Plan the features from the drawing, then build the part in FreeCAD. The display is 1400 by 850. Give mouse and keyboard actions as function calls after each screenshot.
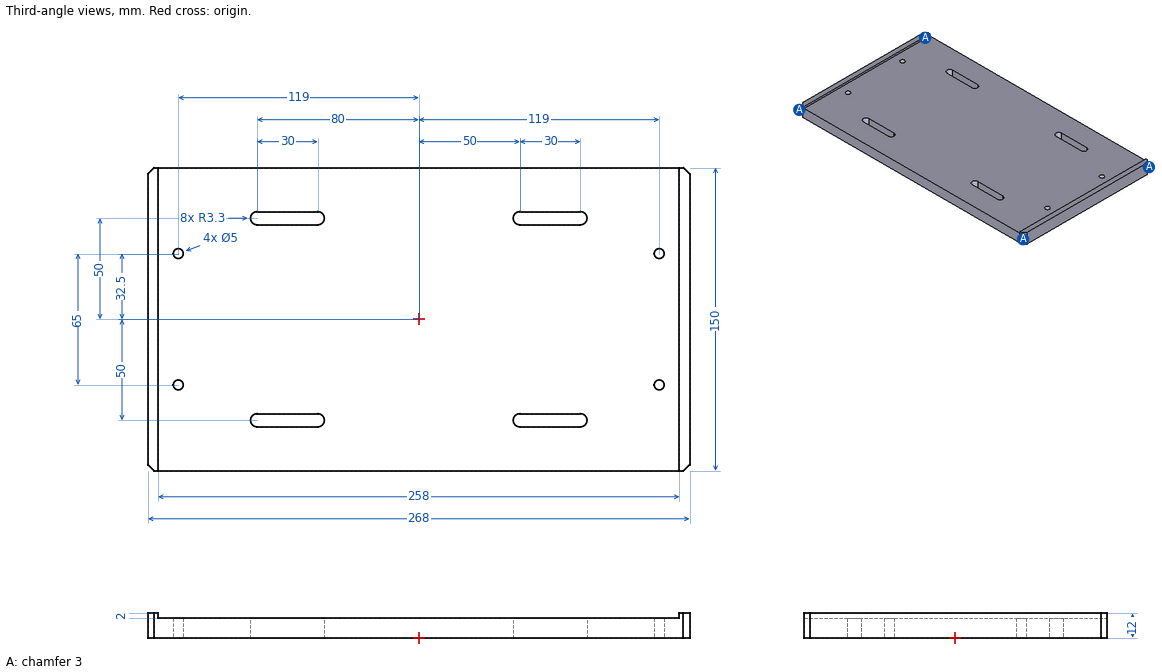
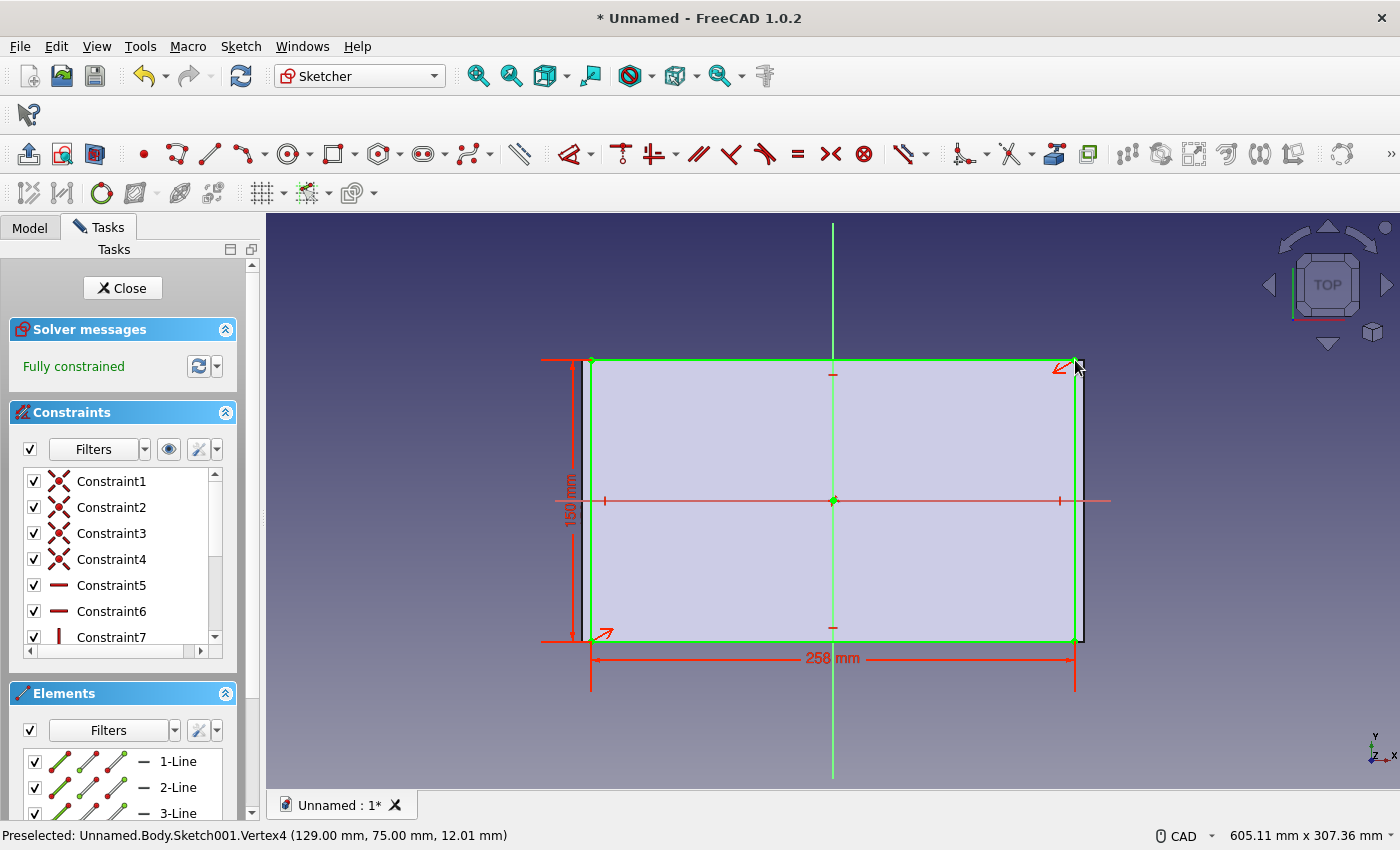
click(123, 288)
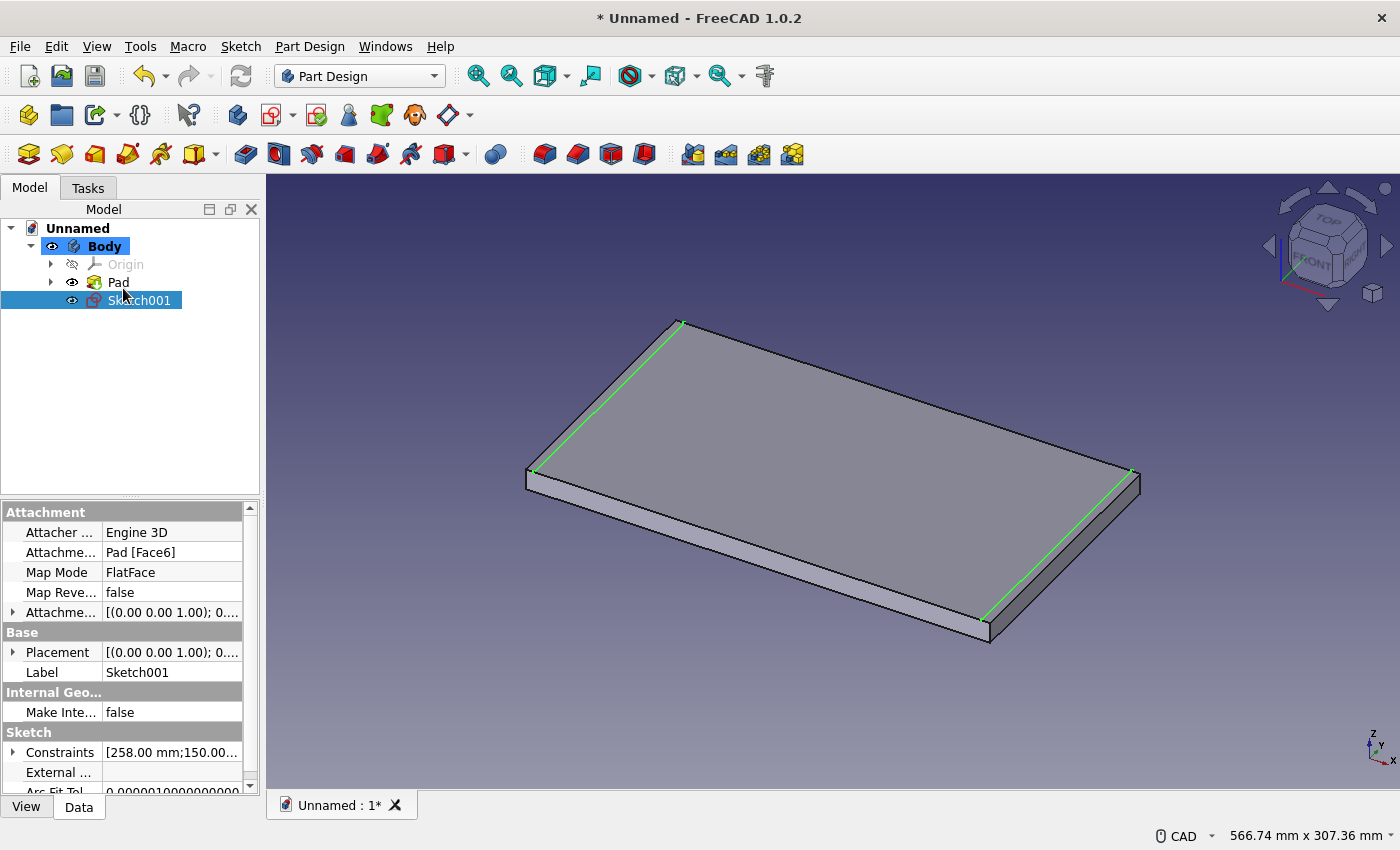
click(246, 154)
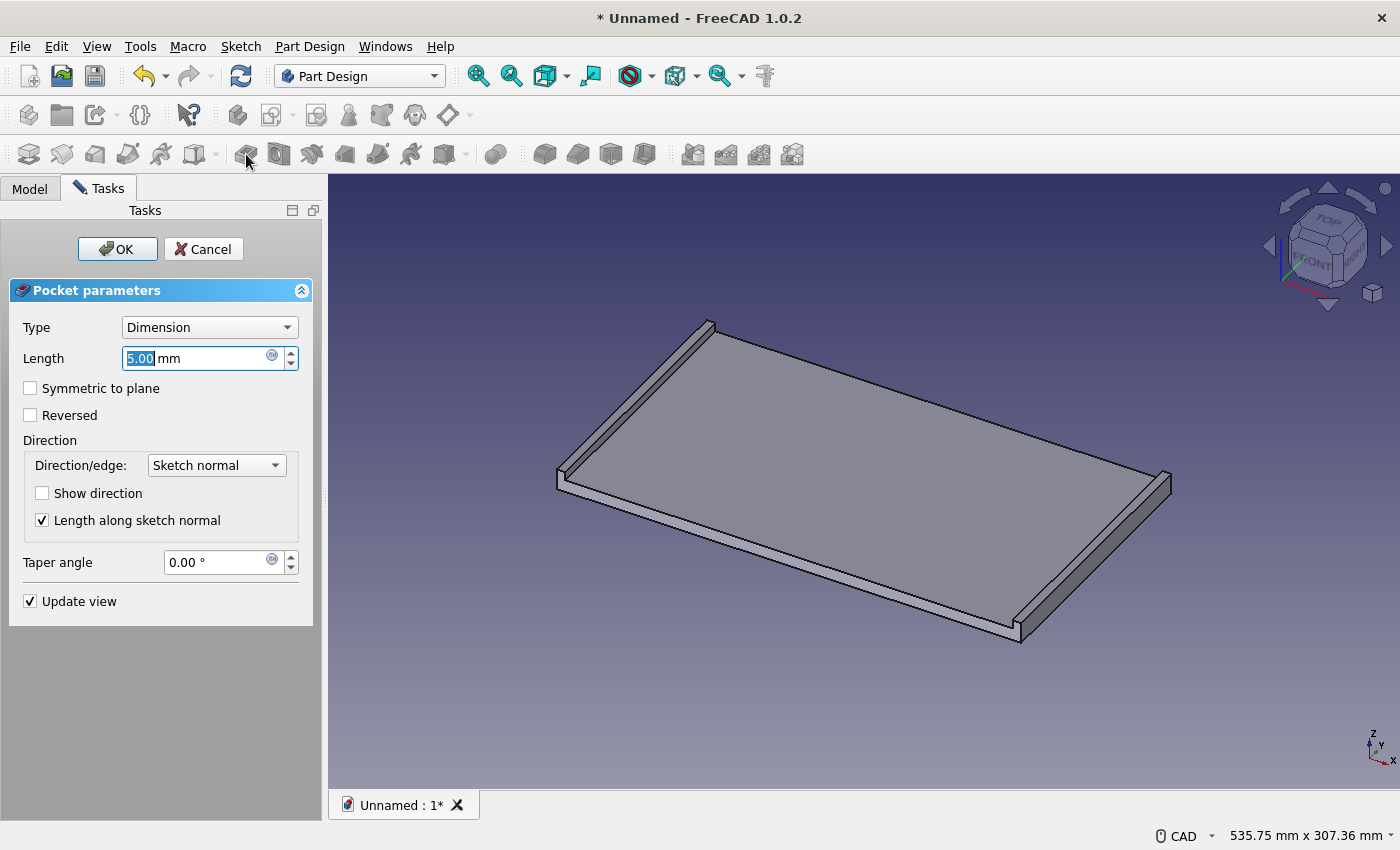
text(2)
key(Tab)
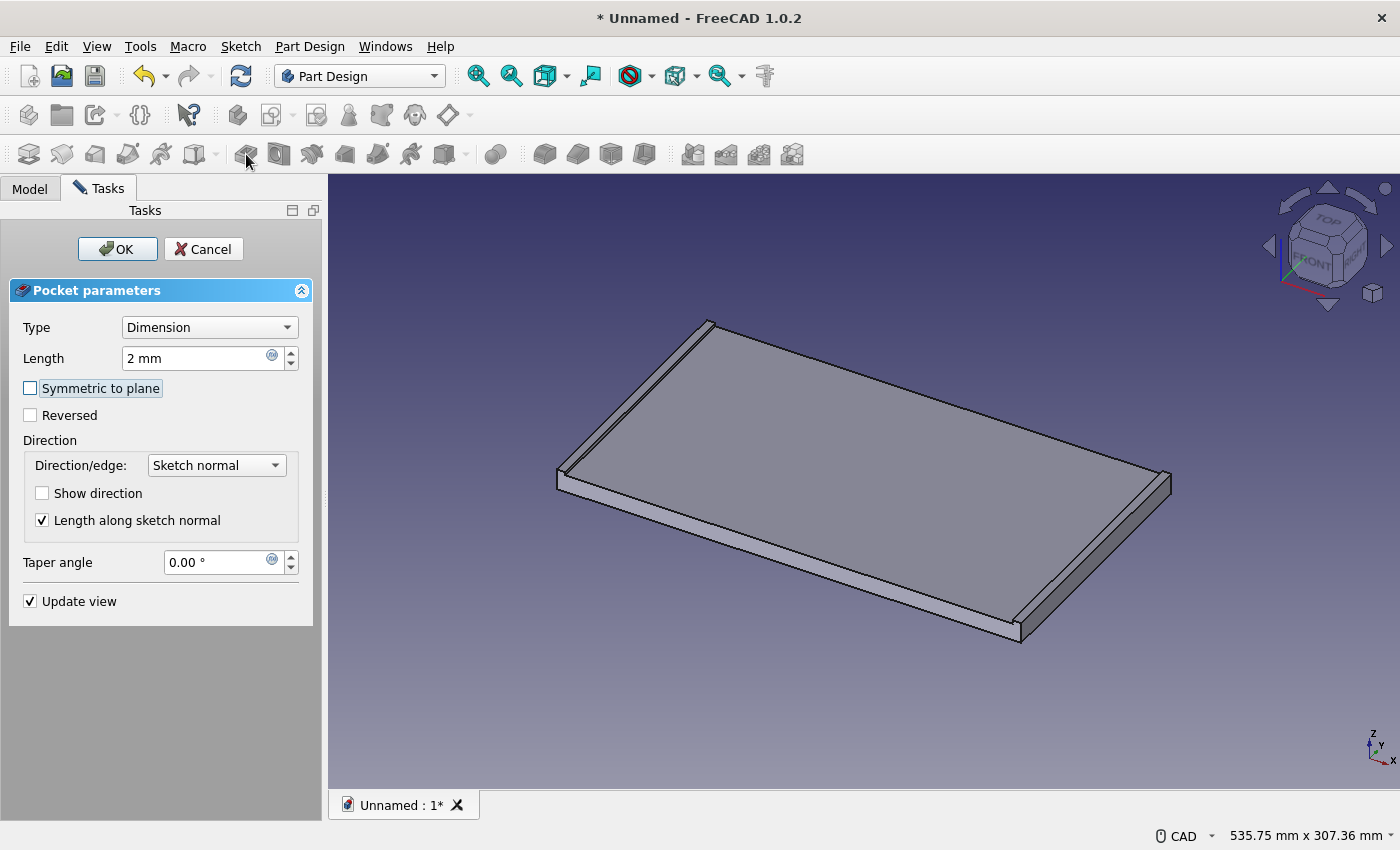
click(118, 249)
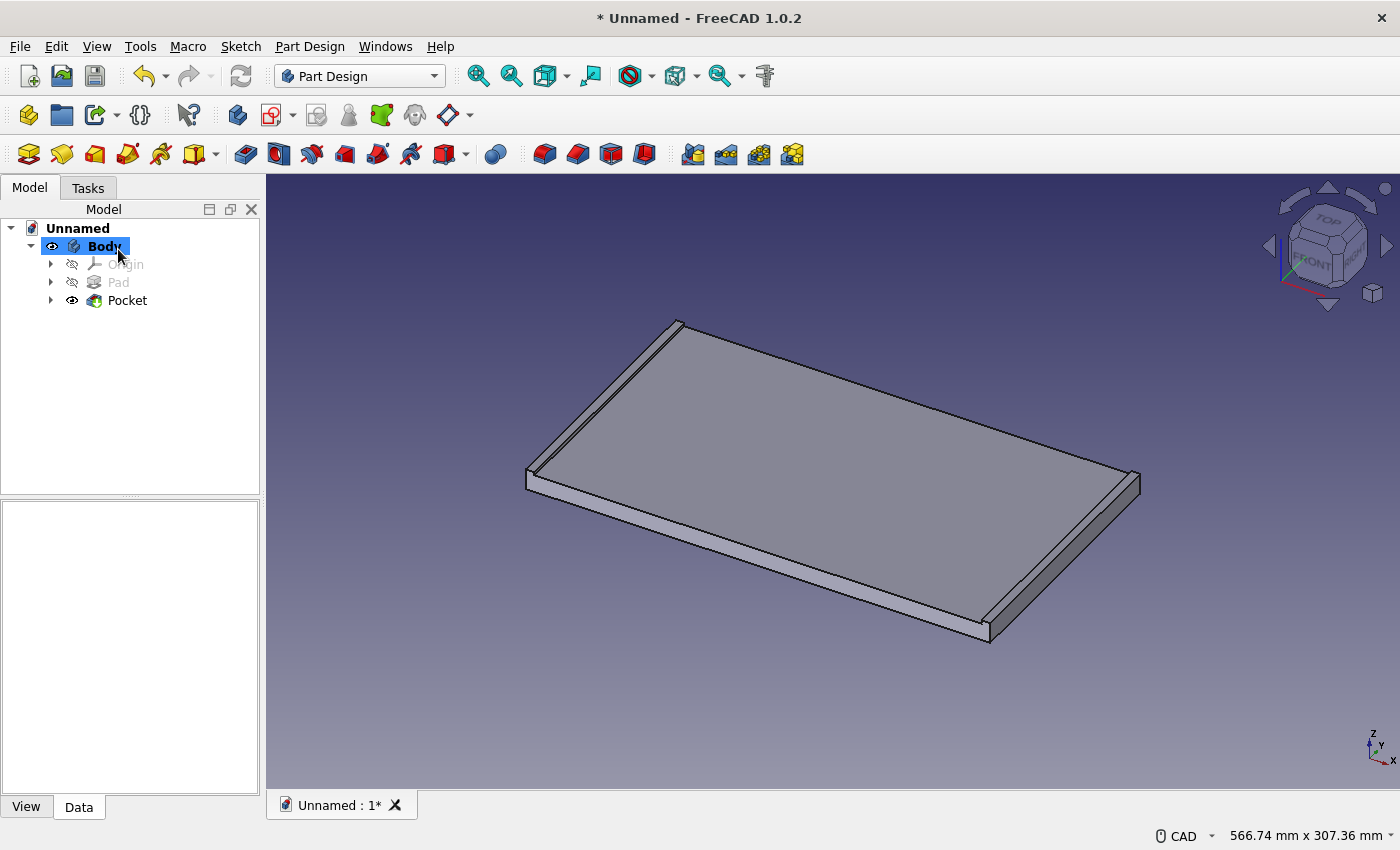
click(897, 495)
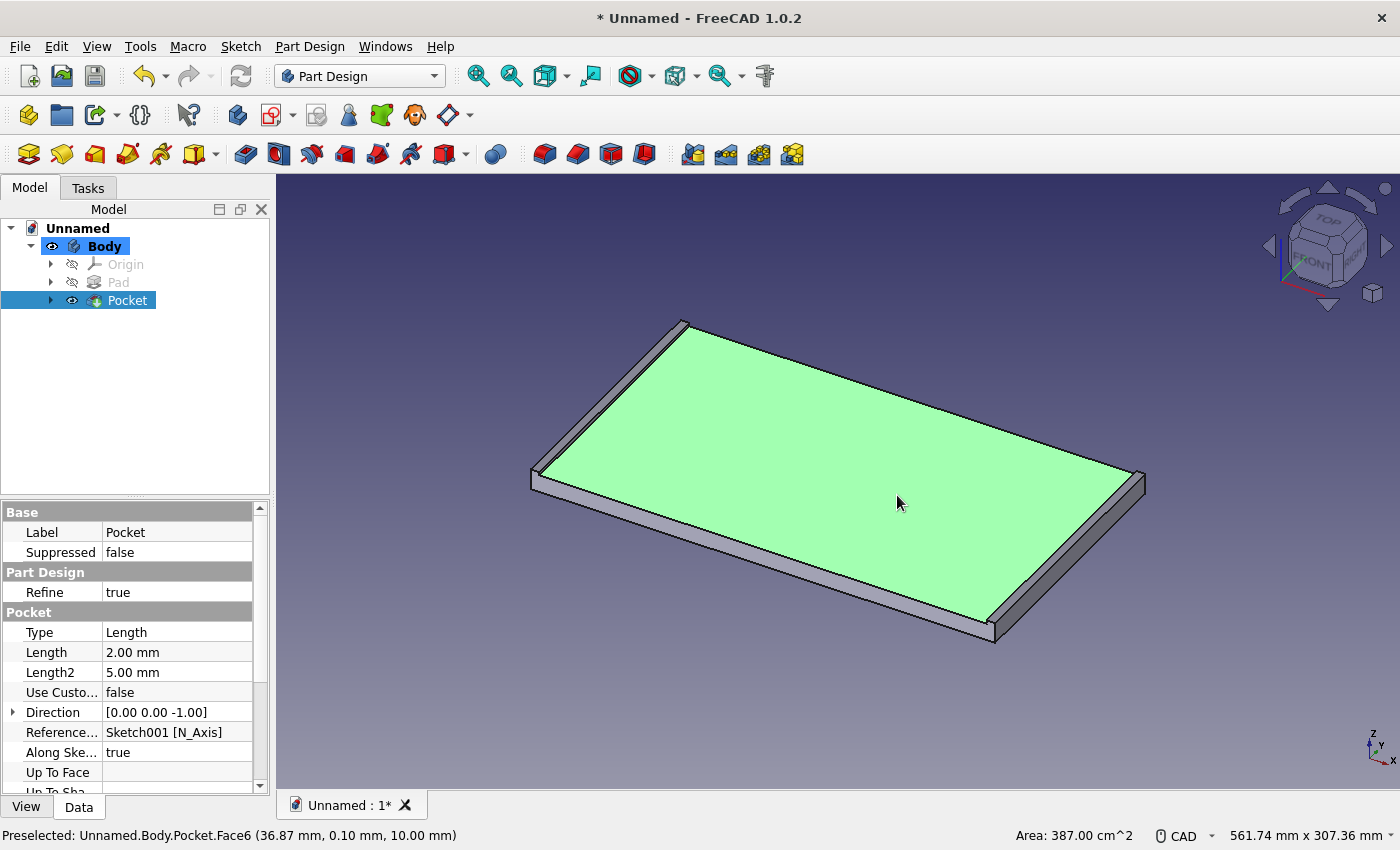
click(270, 116)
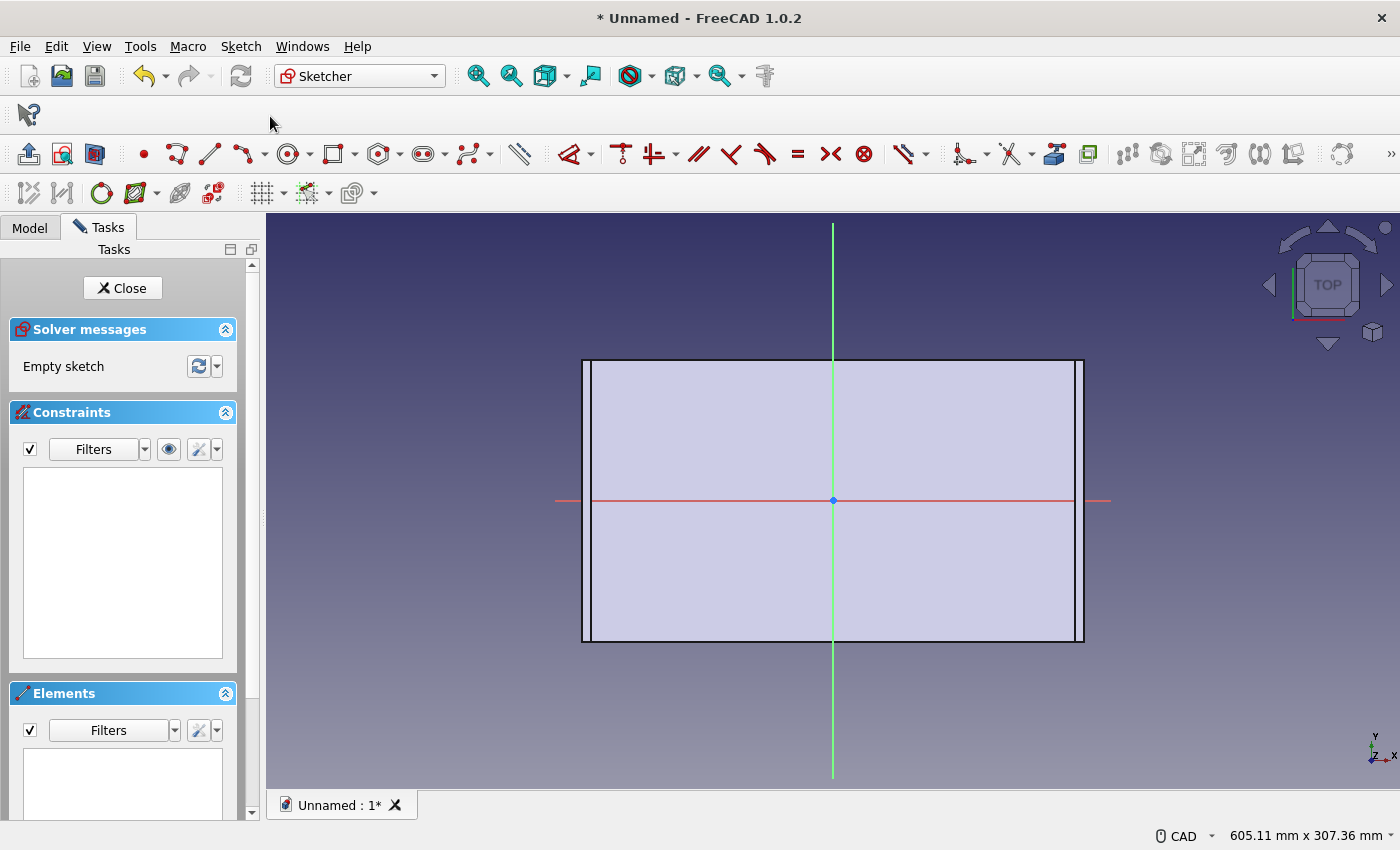
scroll(916, 501, up, 3)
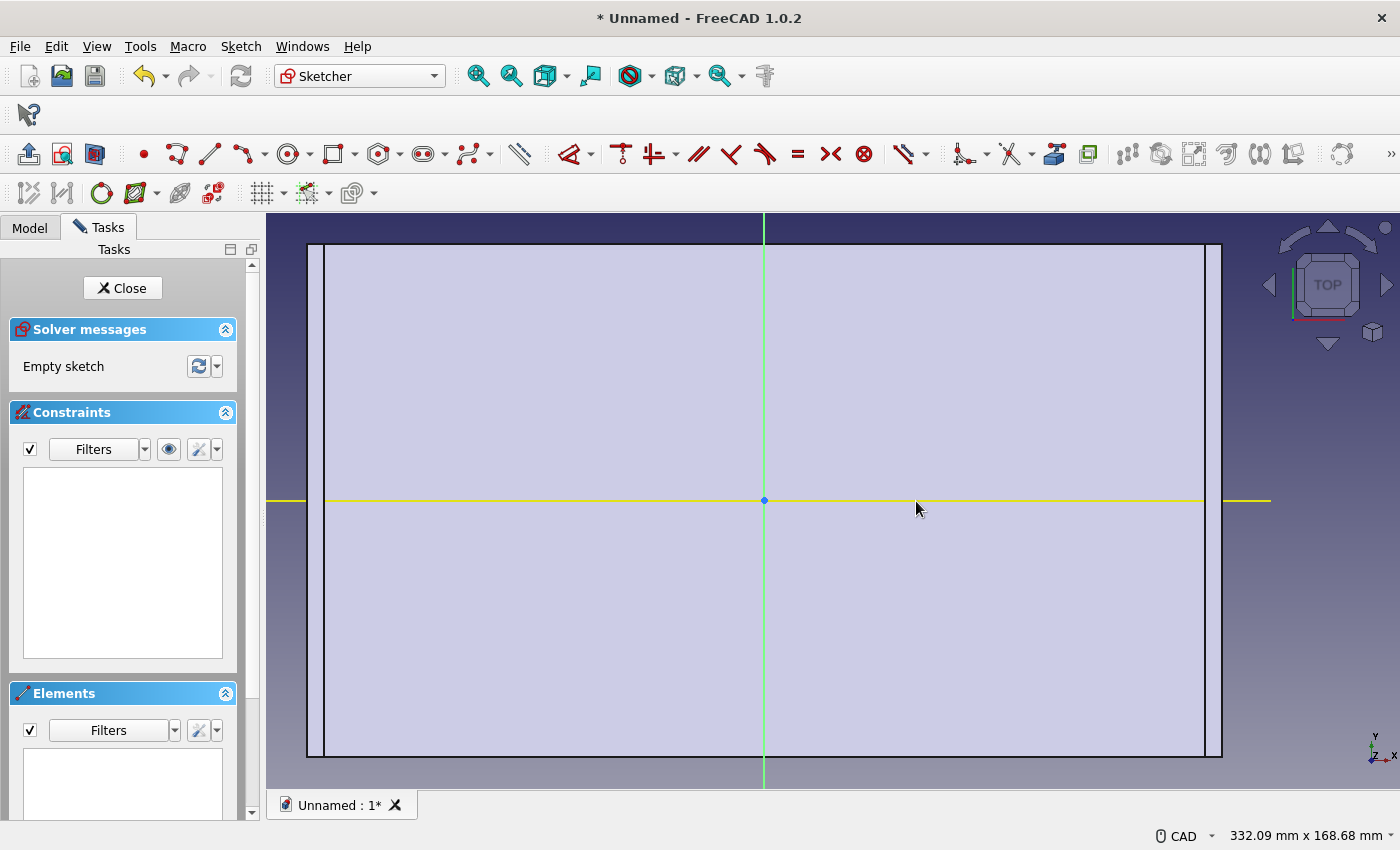
click(422, 154)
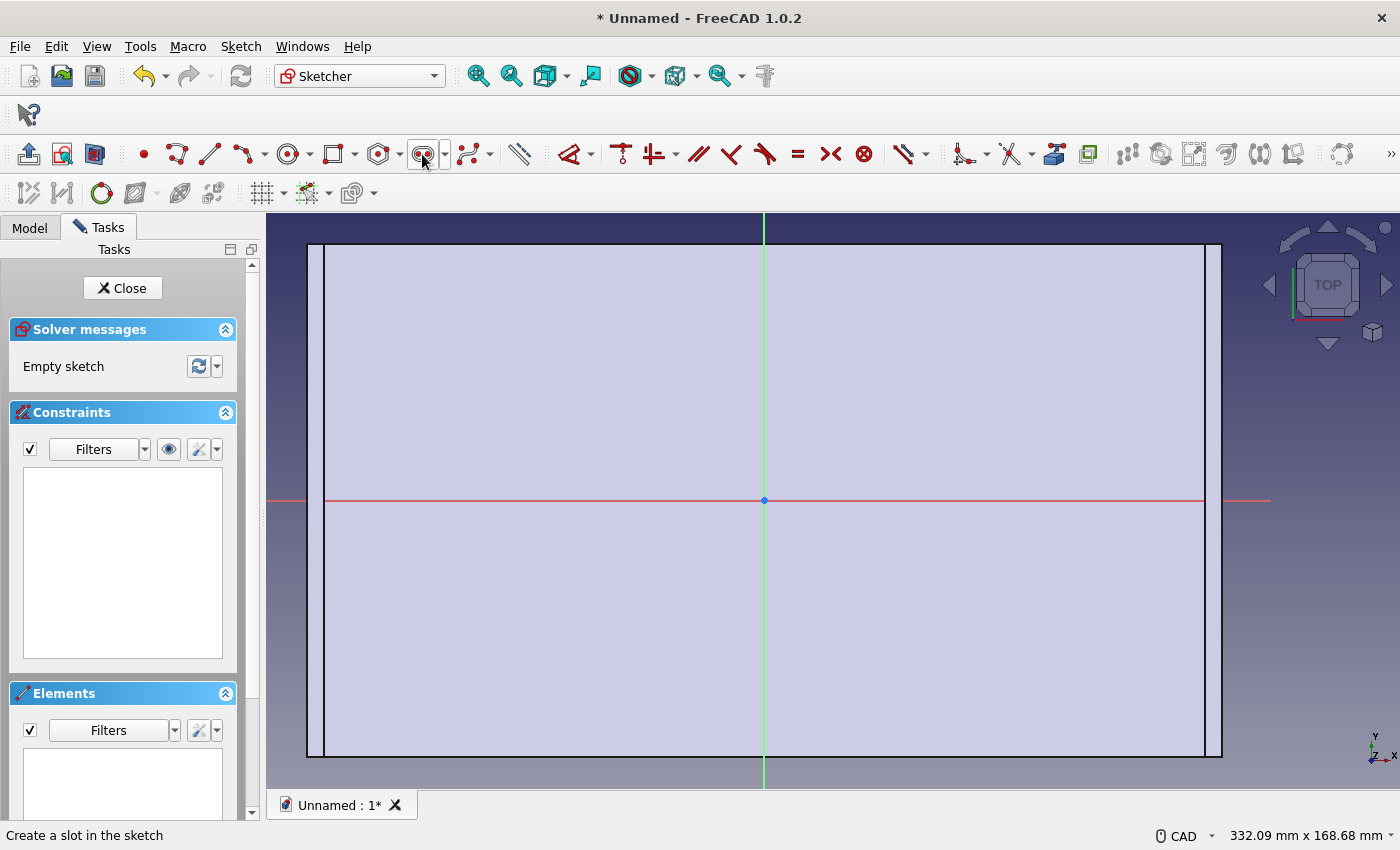
scroll(491, 330, up, 4)